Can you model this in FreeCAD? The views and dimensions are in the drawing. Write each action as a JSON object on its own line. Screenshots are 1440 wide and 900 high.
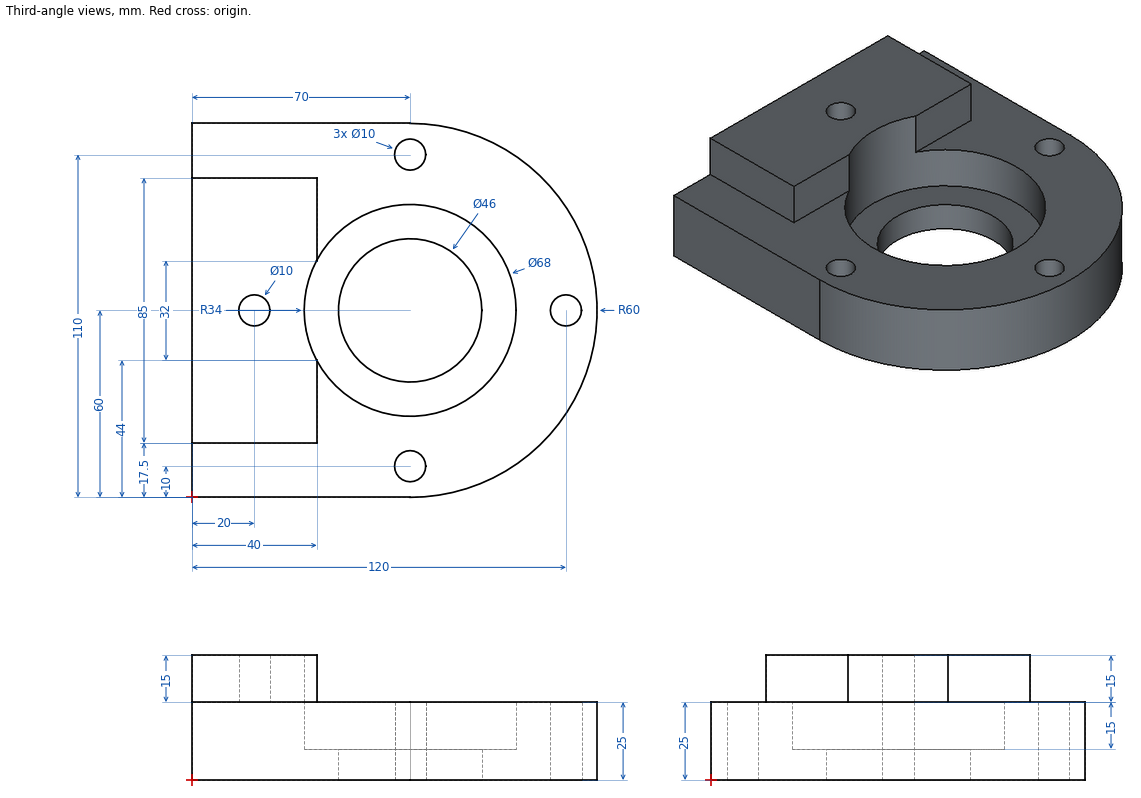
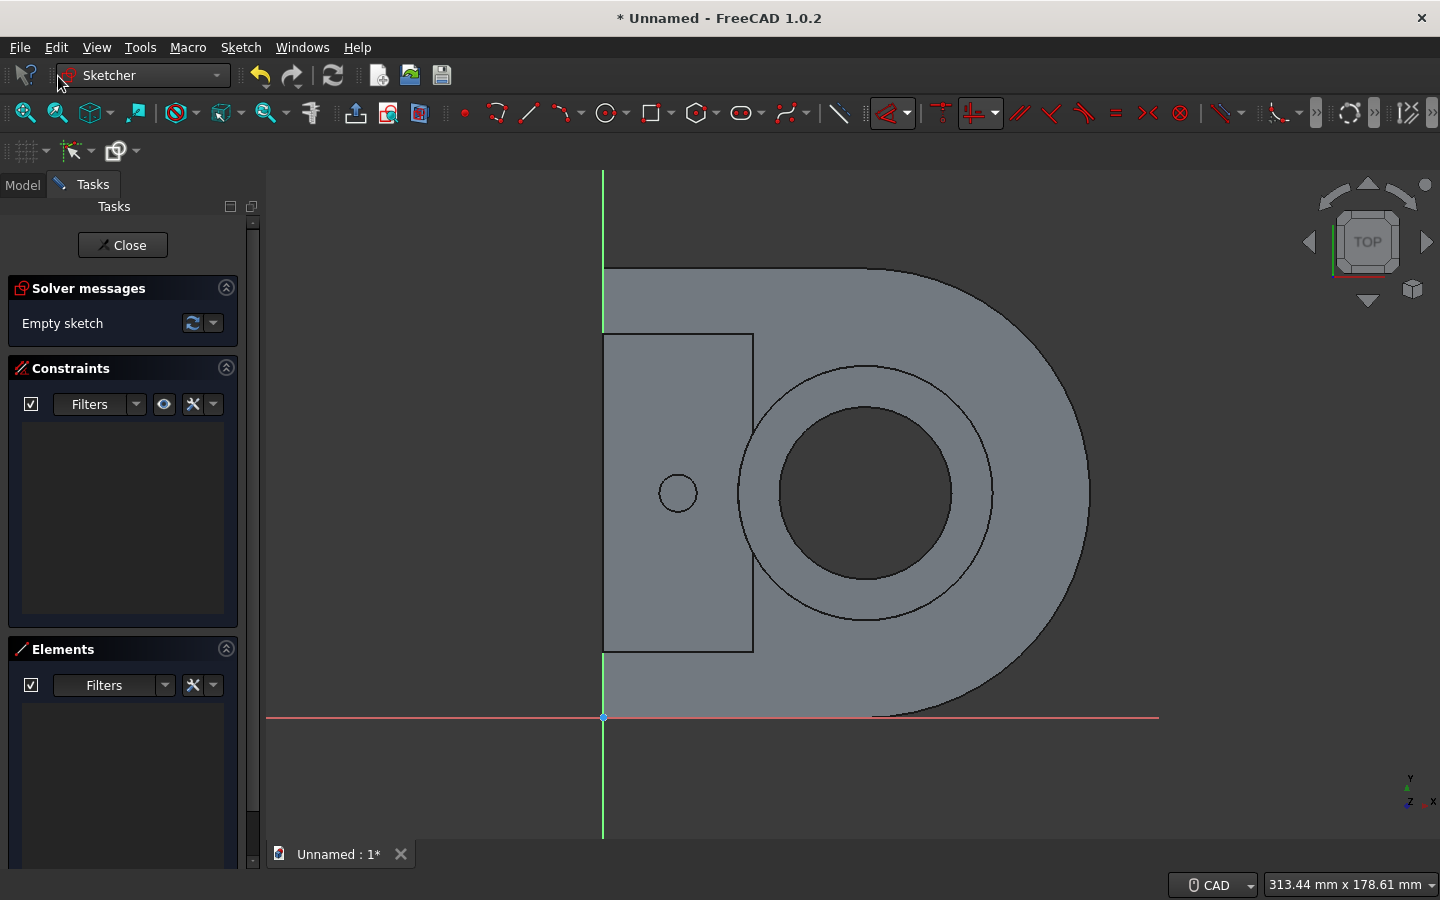
{"action": "left_click", "coordinate": [420, 114]}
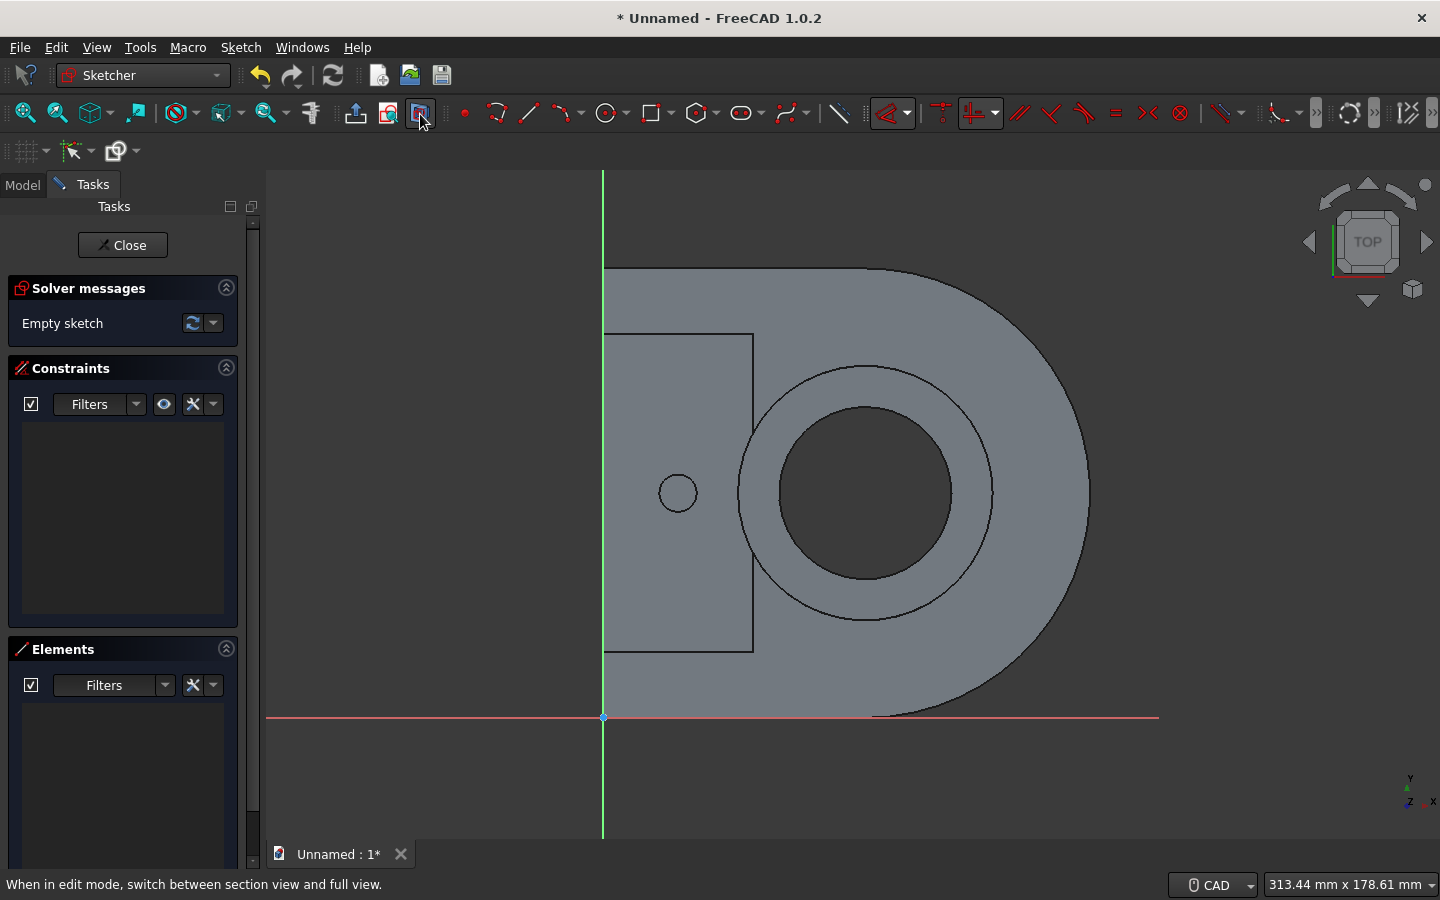
{"action": "left_click", "coordinate": [606, 114]}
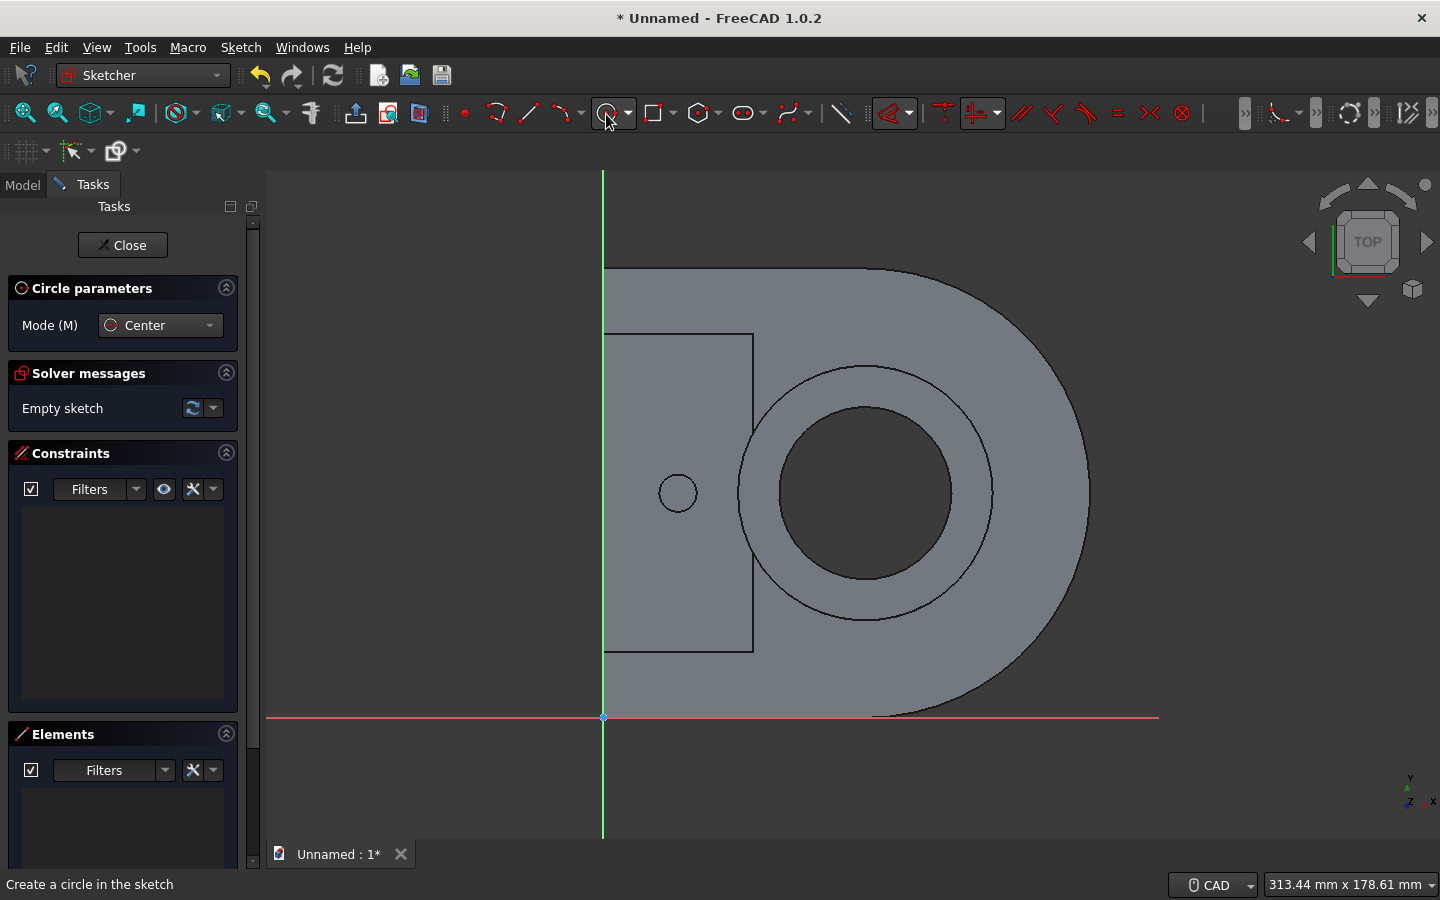
{"action": "left_click", "coordinate": [865, 306]}
{"action": "left_click", "coordinate": [879, 293]}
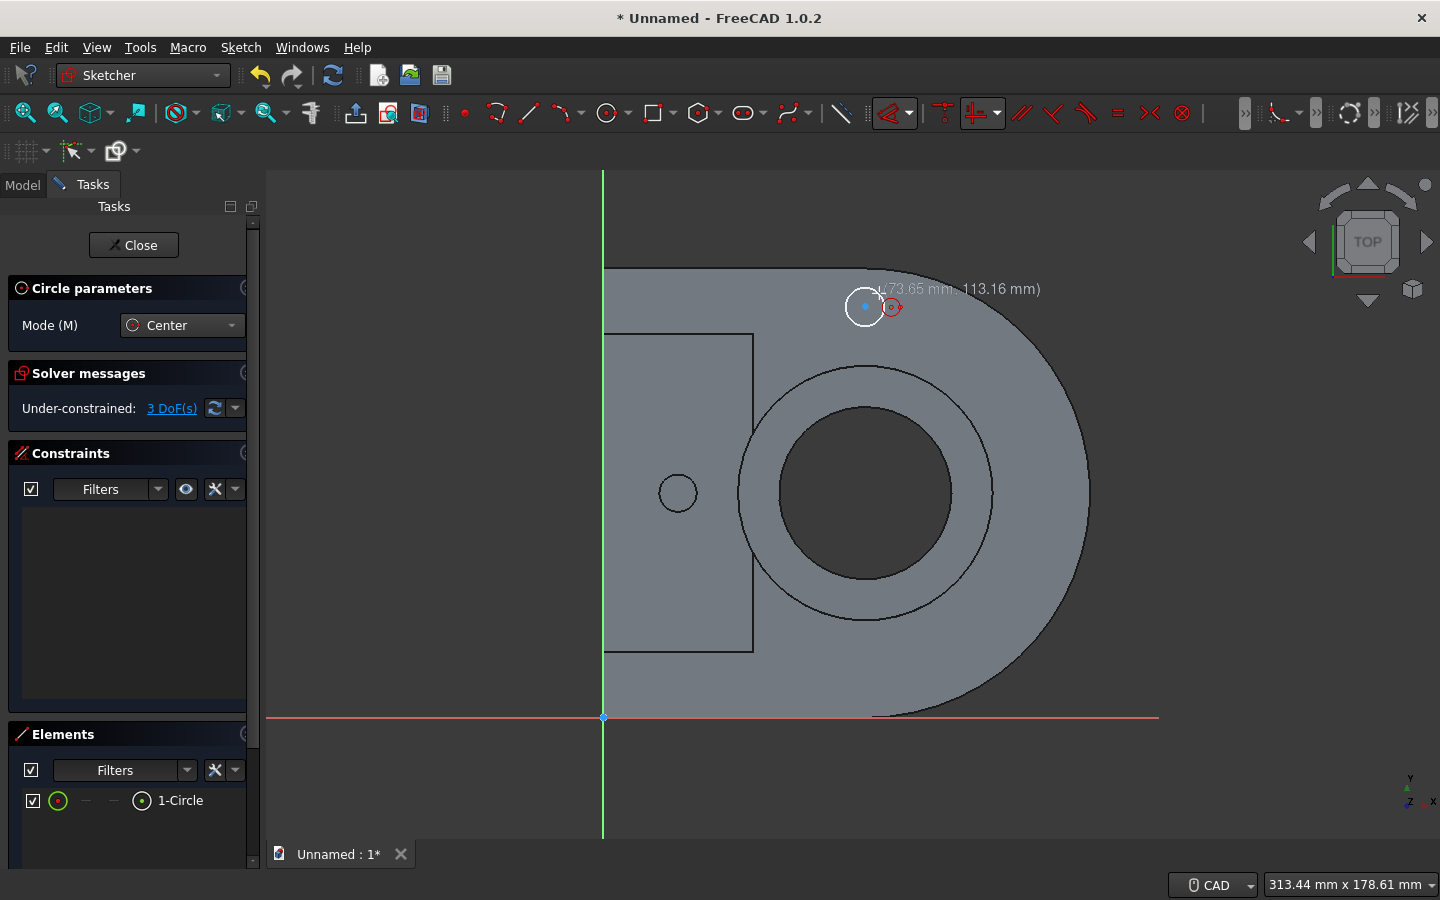
{"action": "left_click", "coordinate": [1053, 493]}
{"action": "left_click", "coordinate": [1066, 480]}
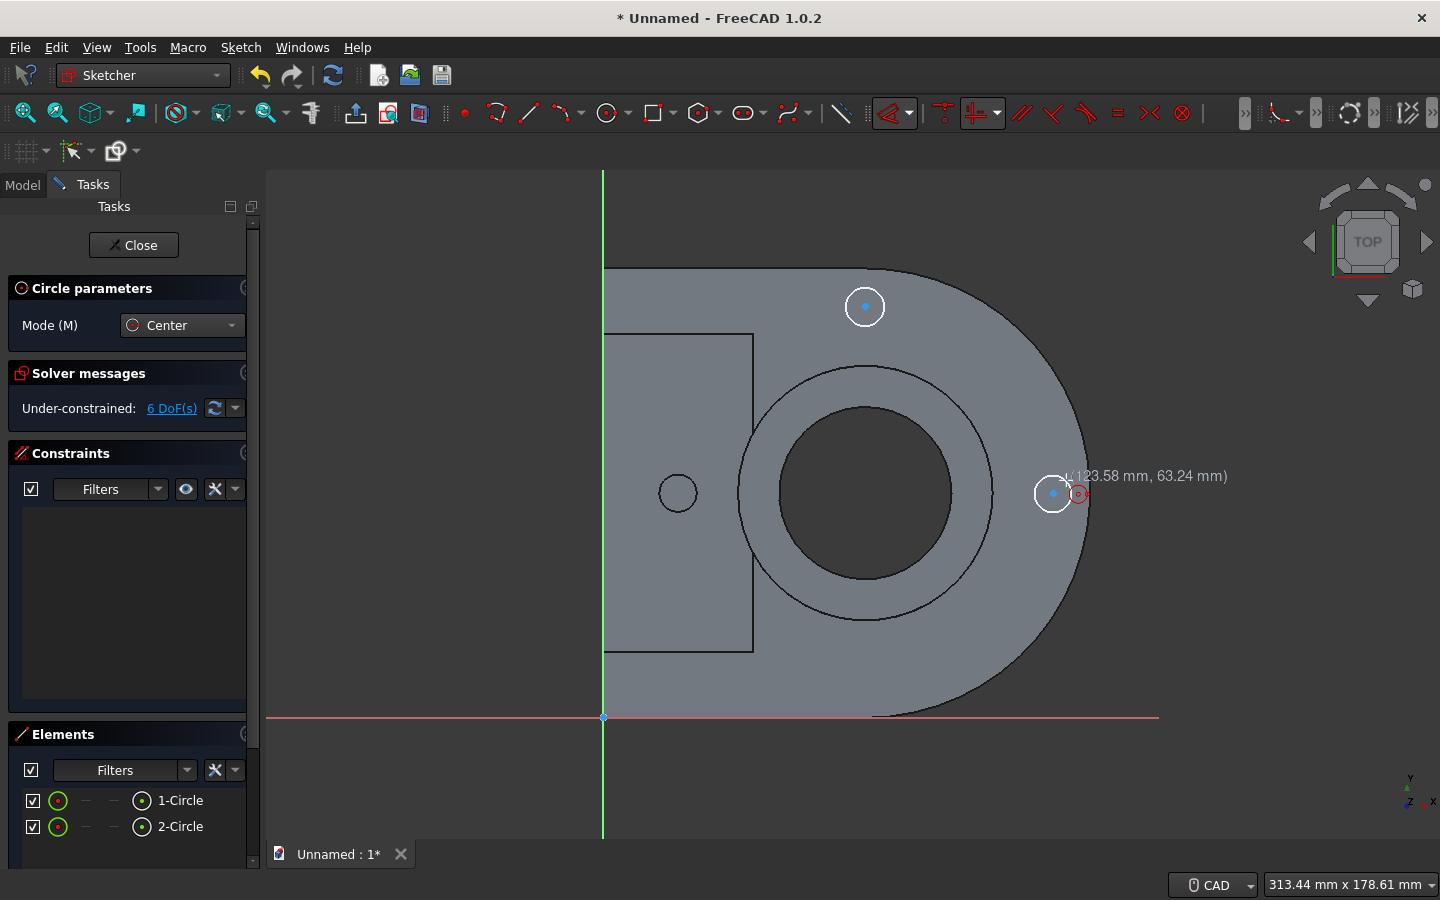
{"action": "left_click", "coordinate": [865, 680]}
{"action": "left_click", "coordinate": [879, 667]}
{"action": "key", "text": "Escape"}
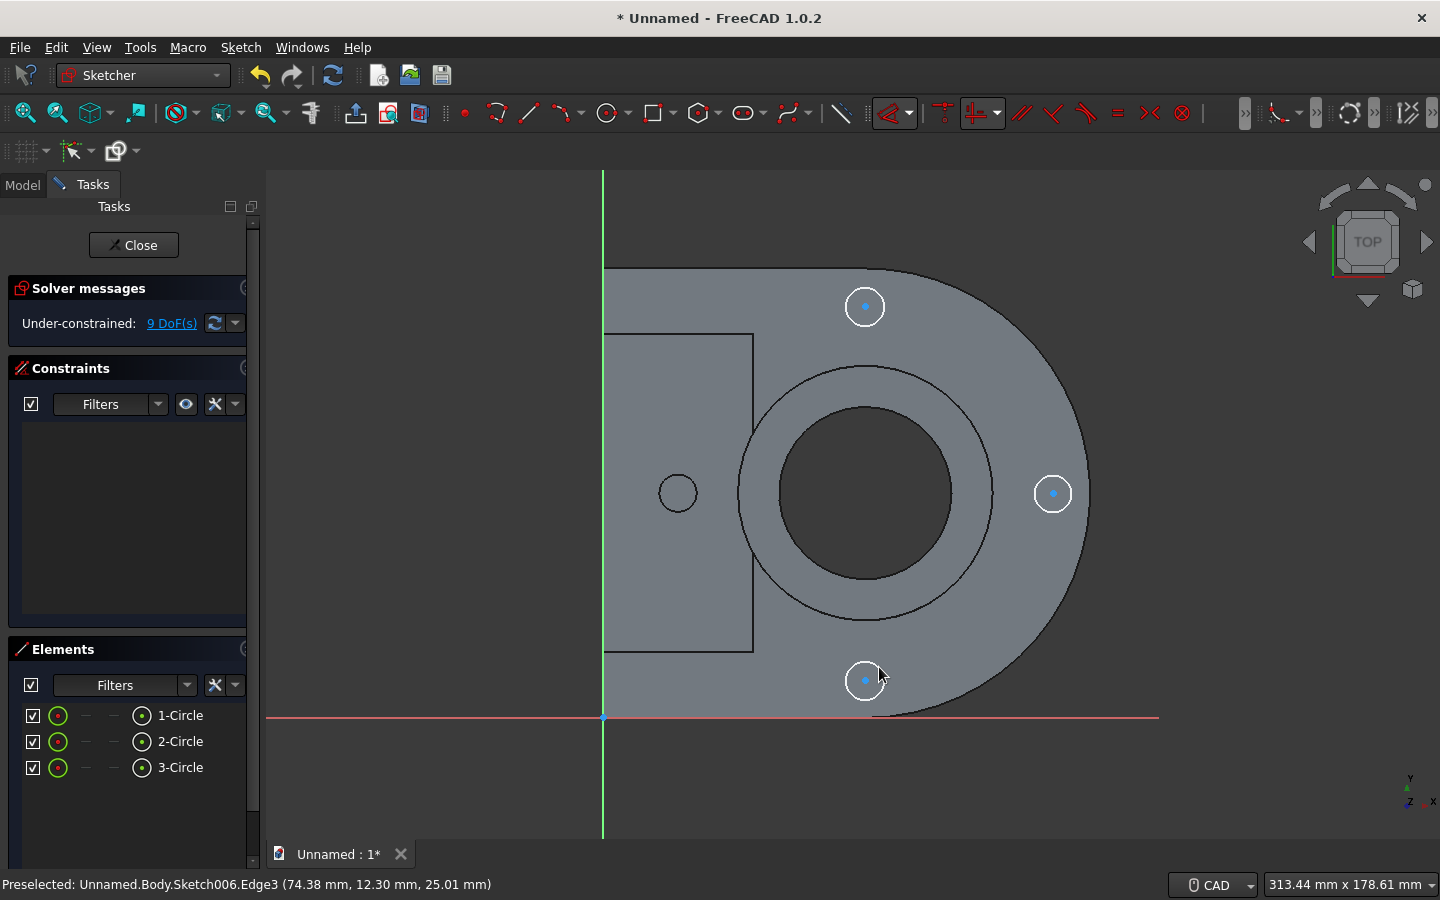
{"action": "left_click", "coordinate": [878, 293]}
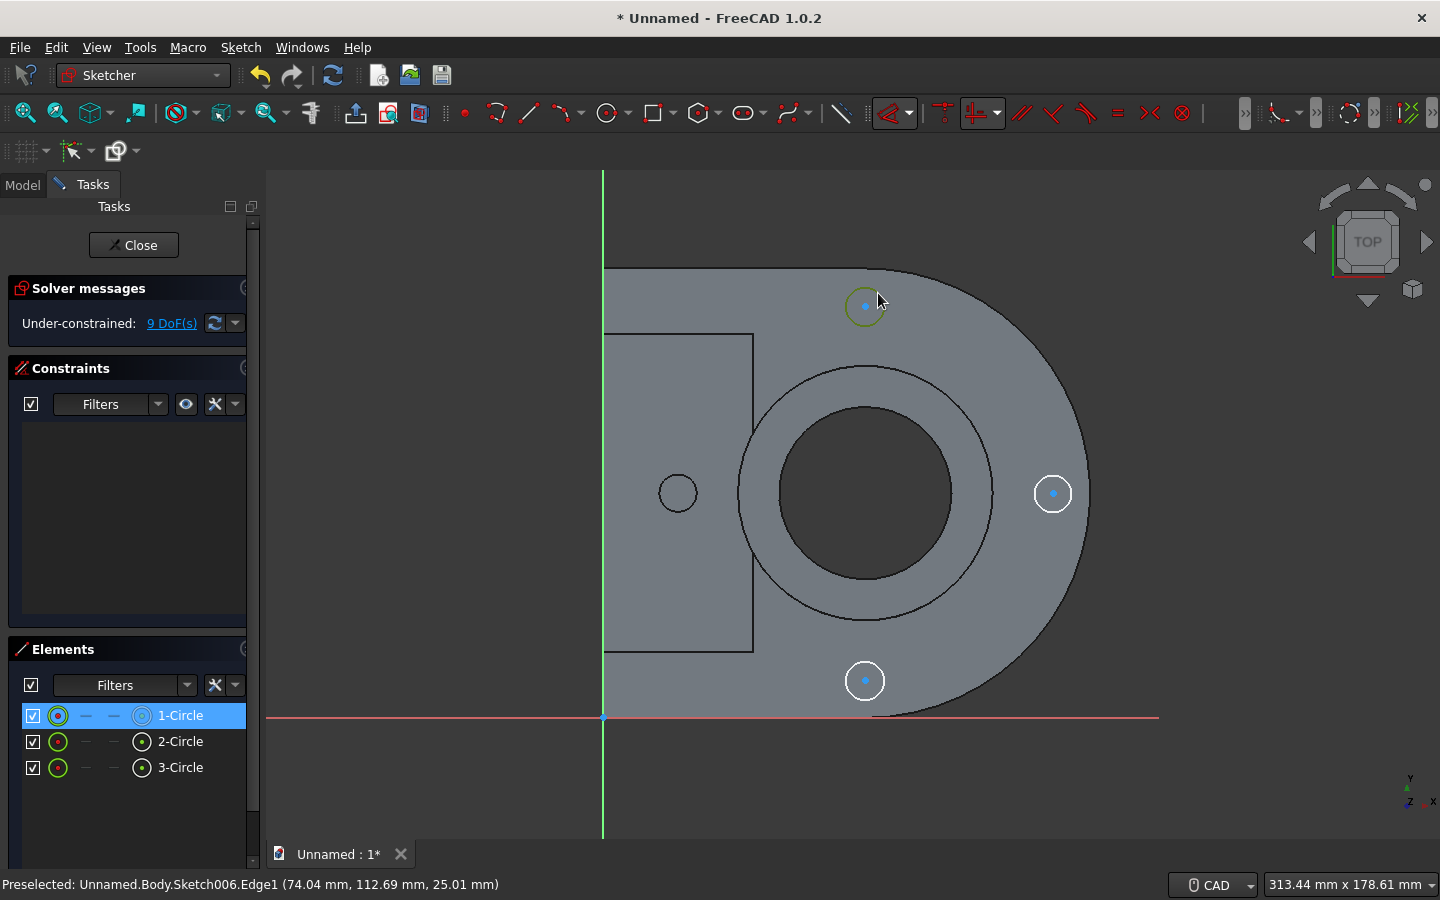
{"action": "left_click", "coordinate": [1066, 481]}